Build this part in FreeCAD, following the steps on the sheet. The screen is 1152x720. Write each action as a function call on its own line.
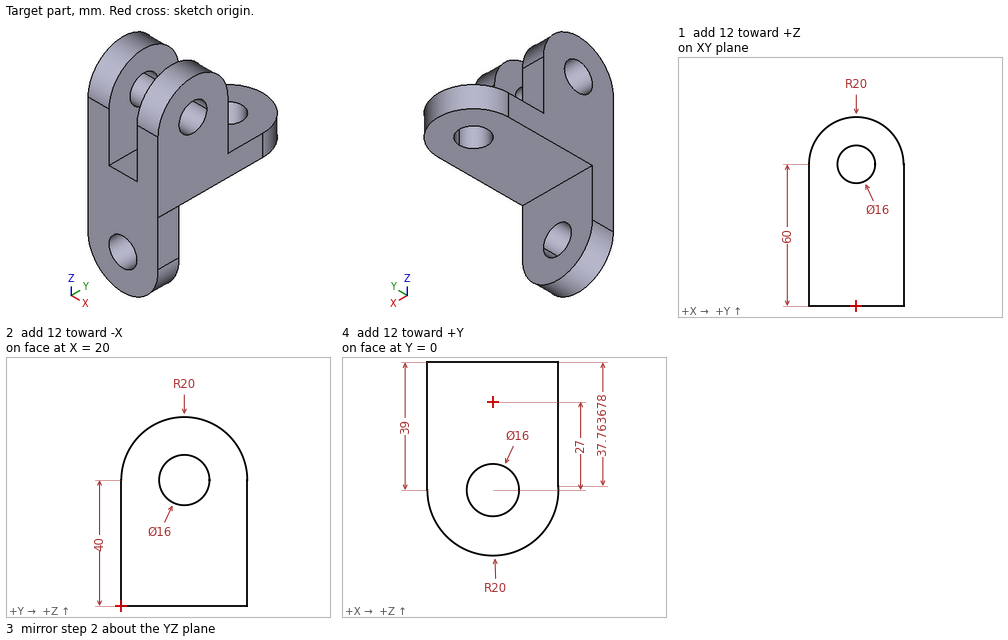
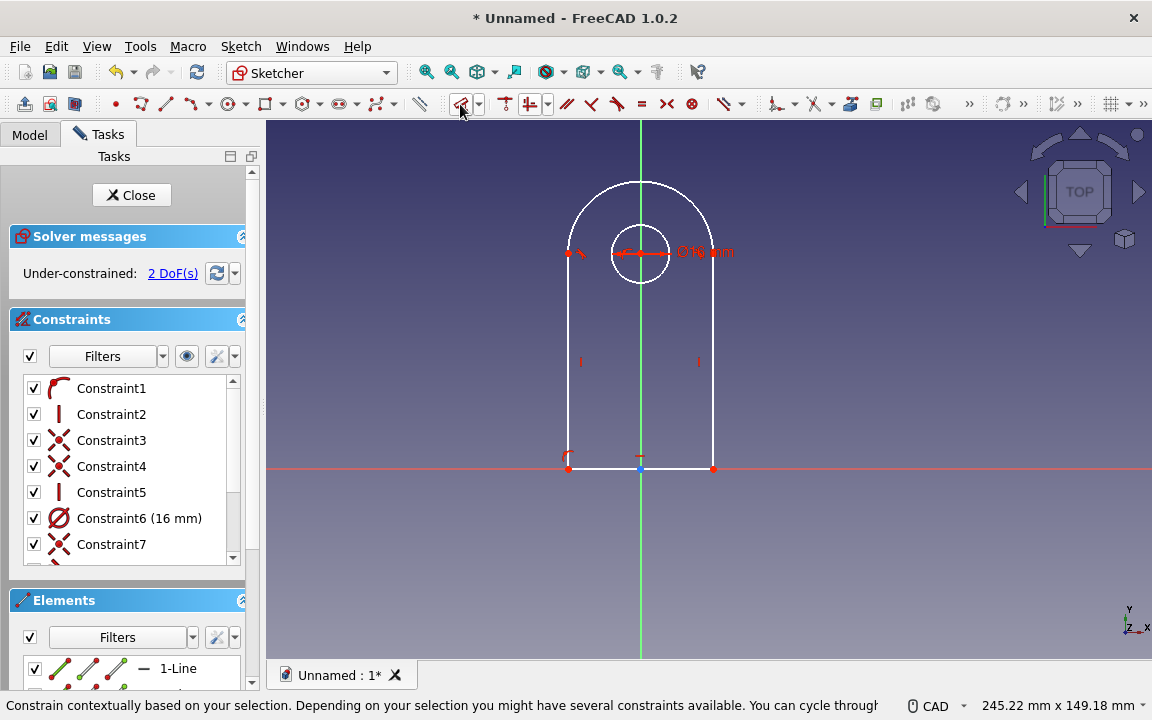
click(683, 195)
click(702, 169)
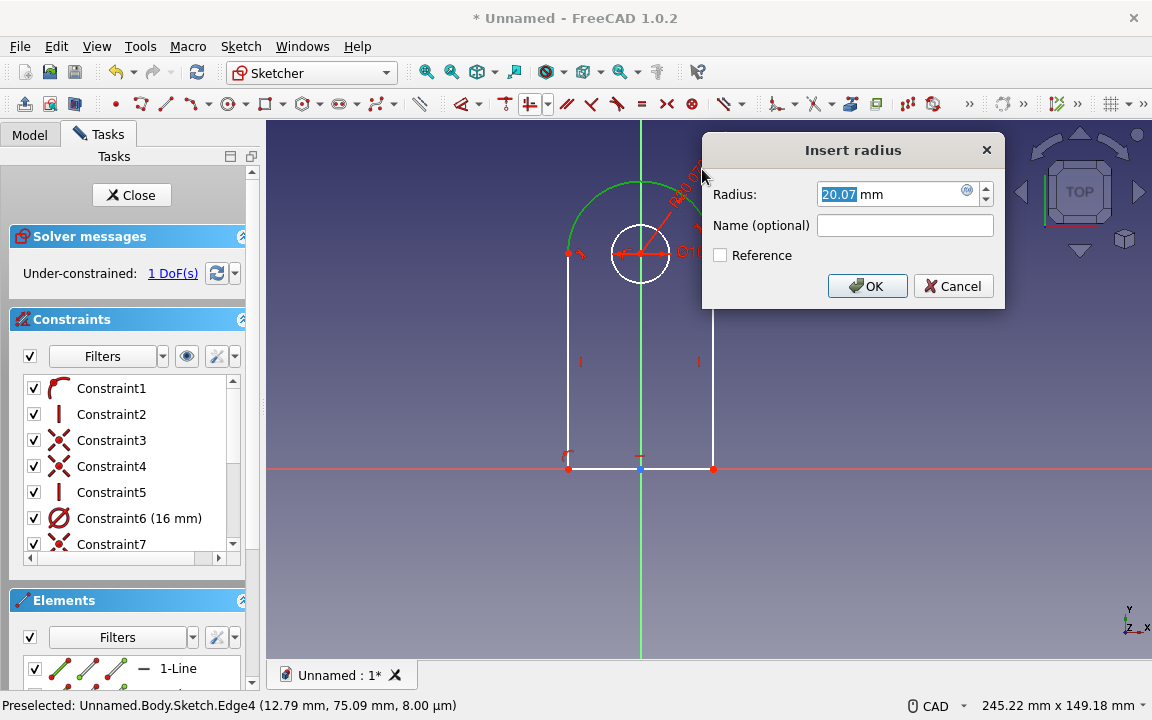
text(20)
key(Return)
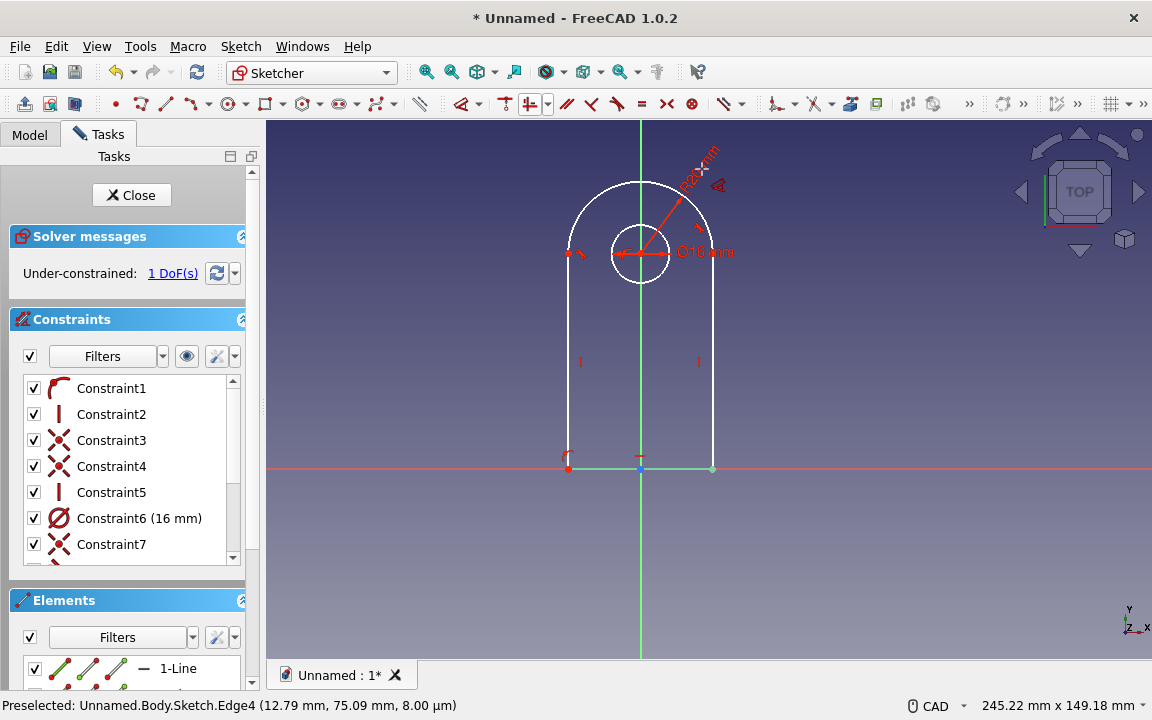
click(568, 319)
click(534, 362)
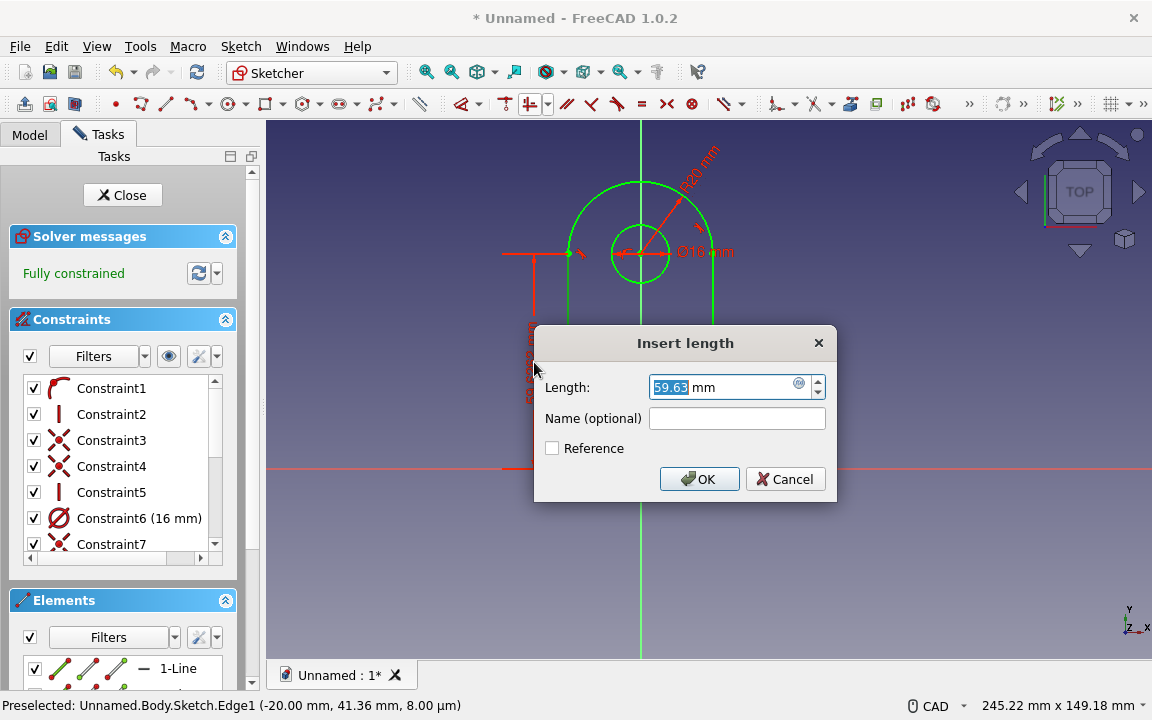
text(60)
key(Return)
key(Escape)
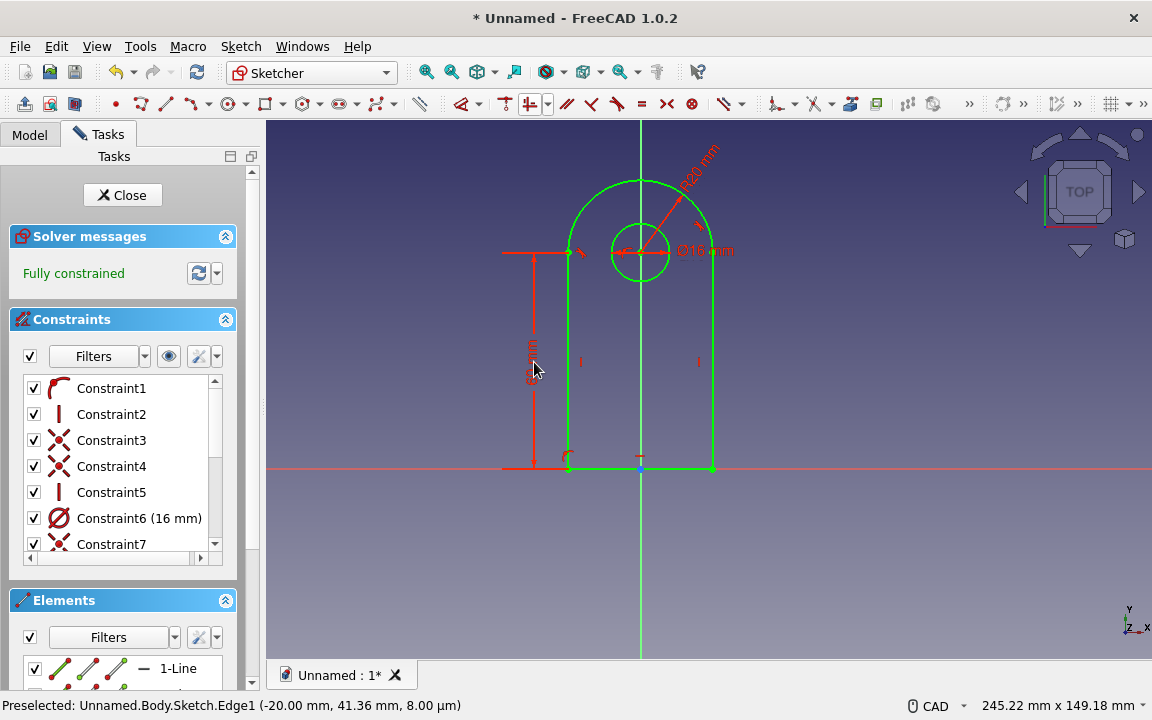
click(123, 195)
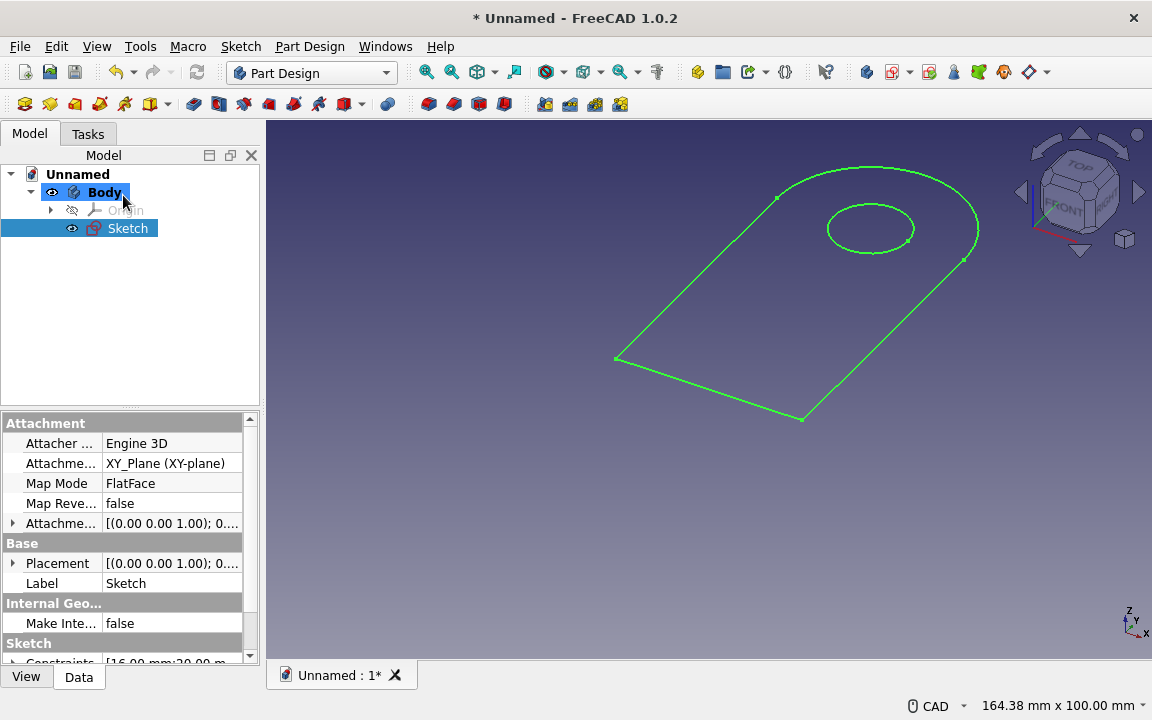
click(25, 104)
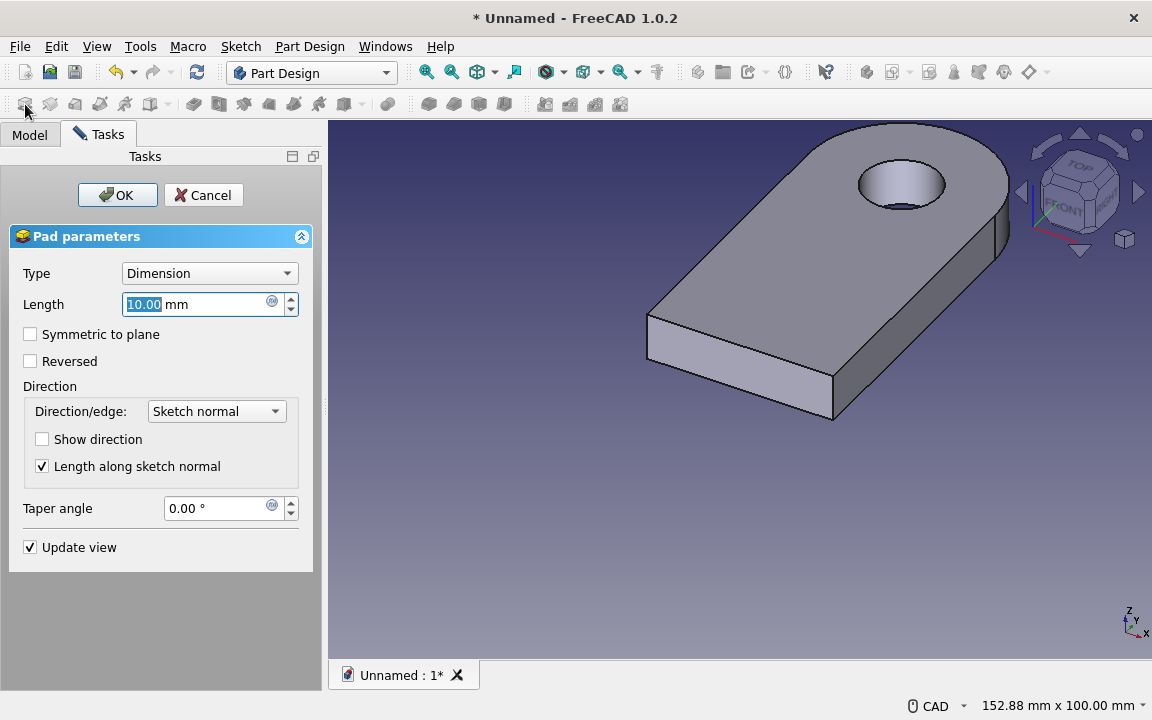
text(12)
key(Tab)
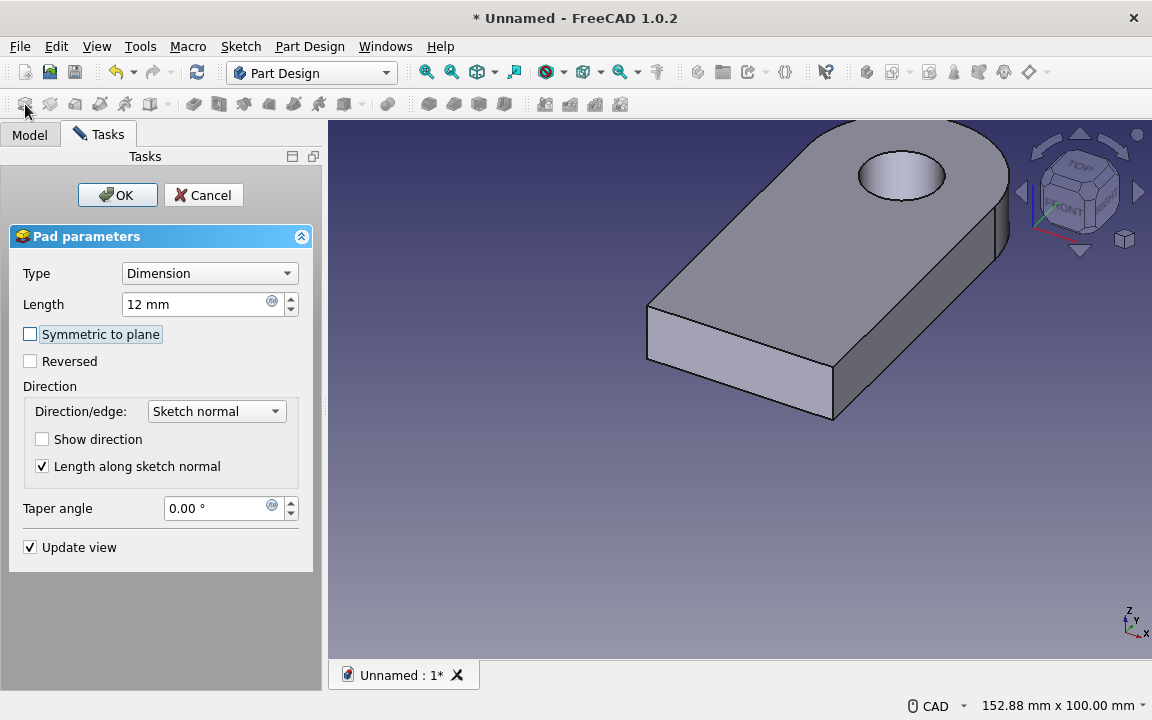
click(118, 195)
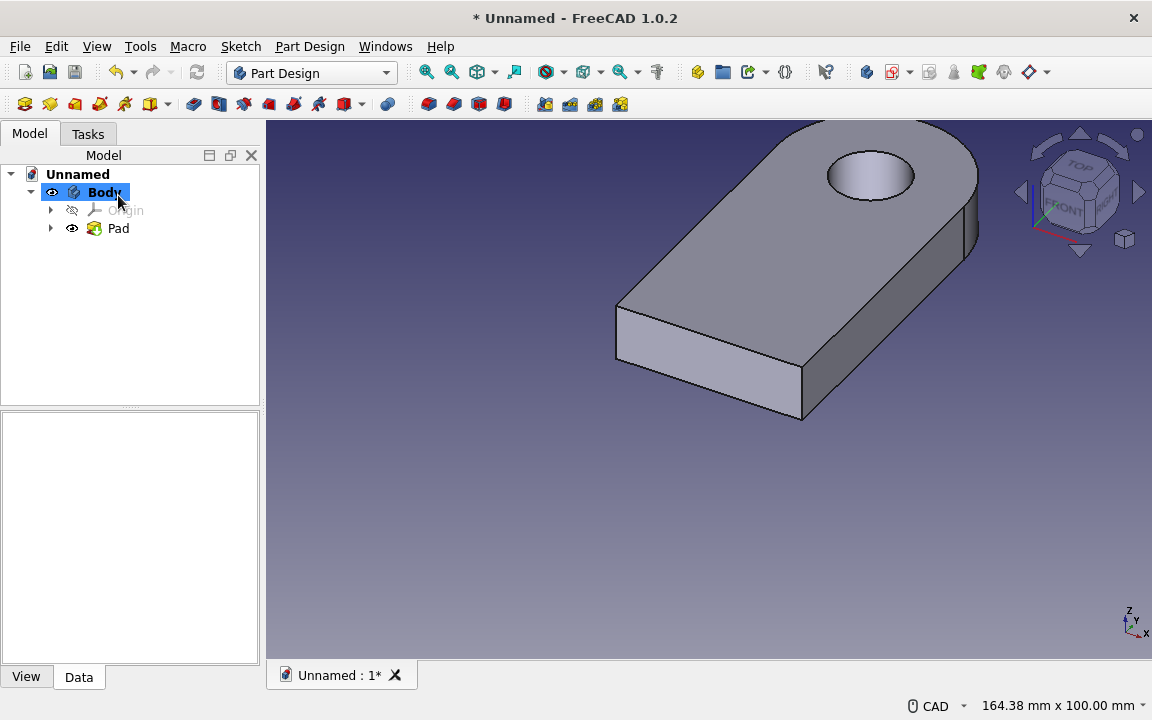
key(v)
key(f)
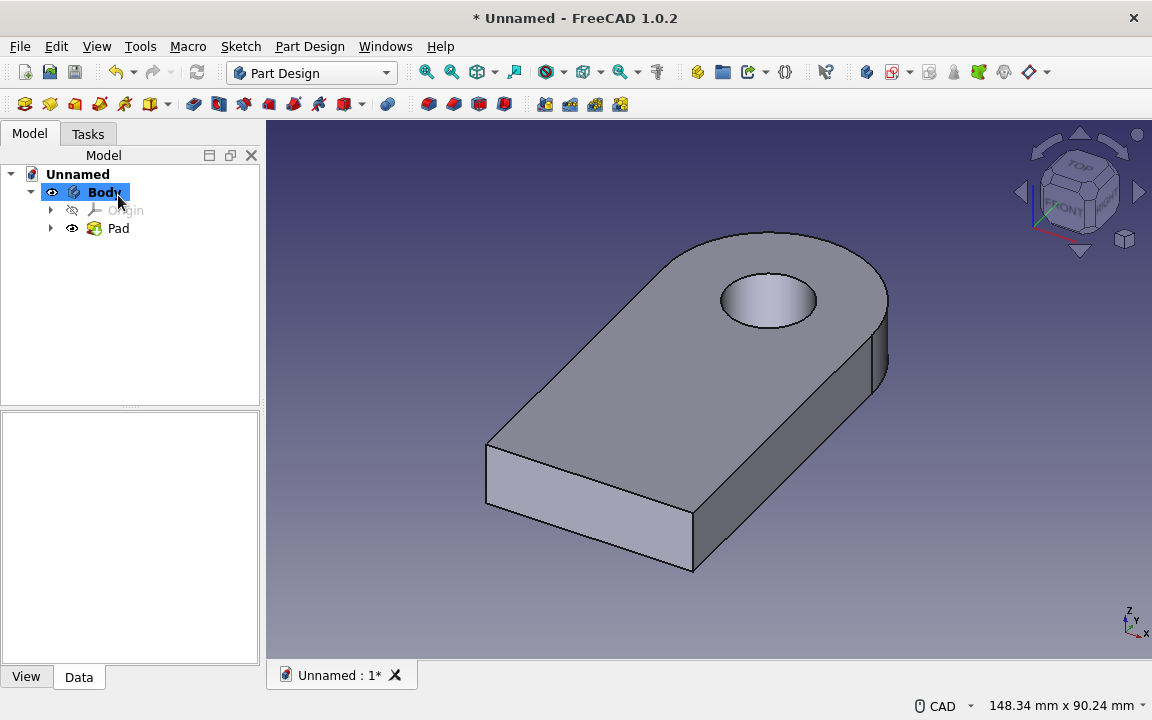
click(834, 402)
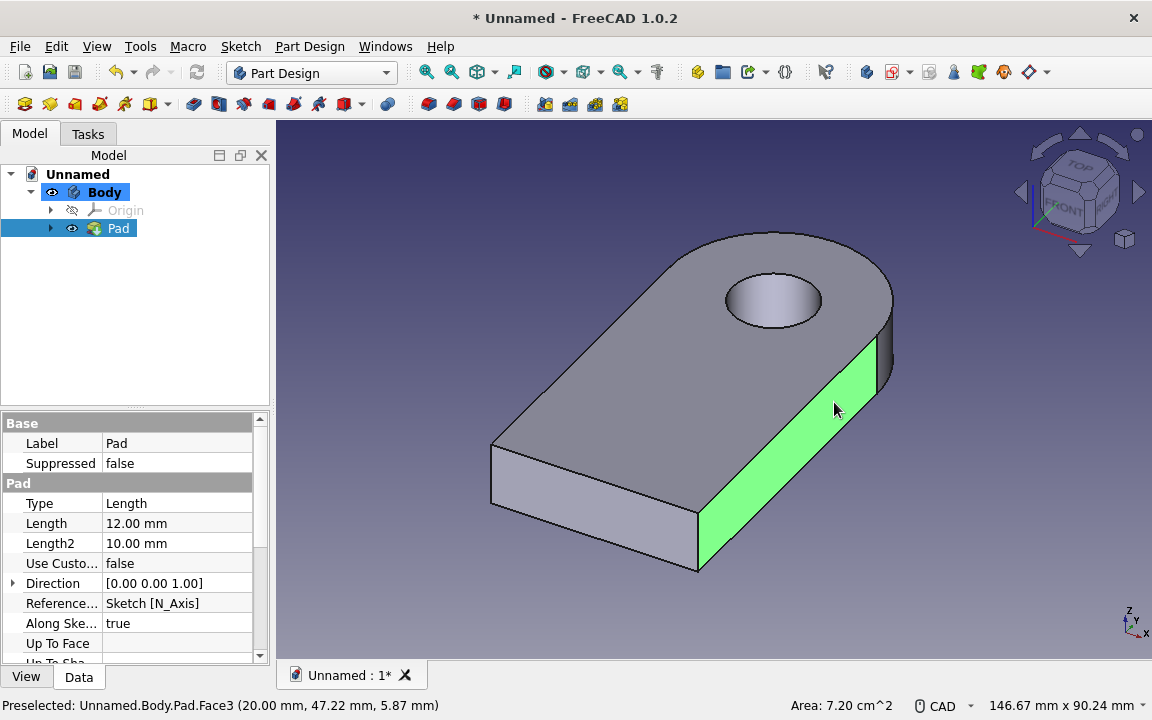
click(892, 72)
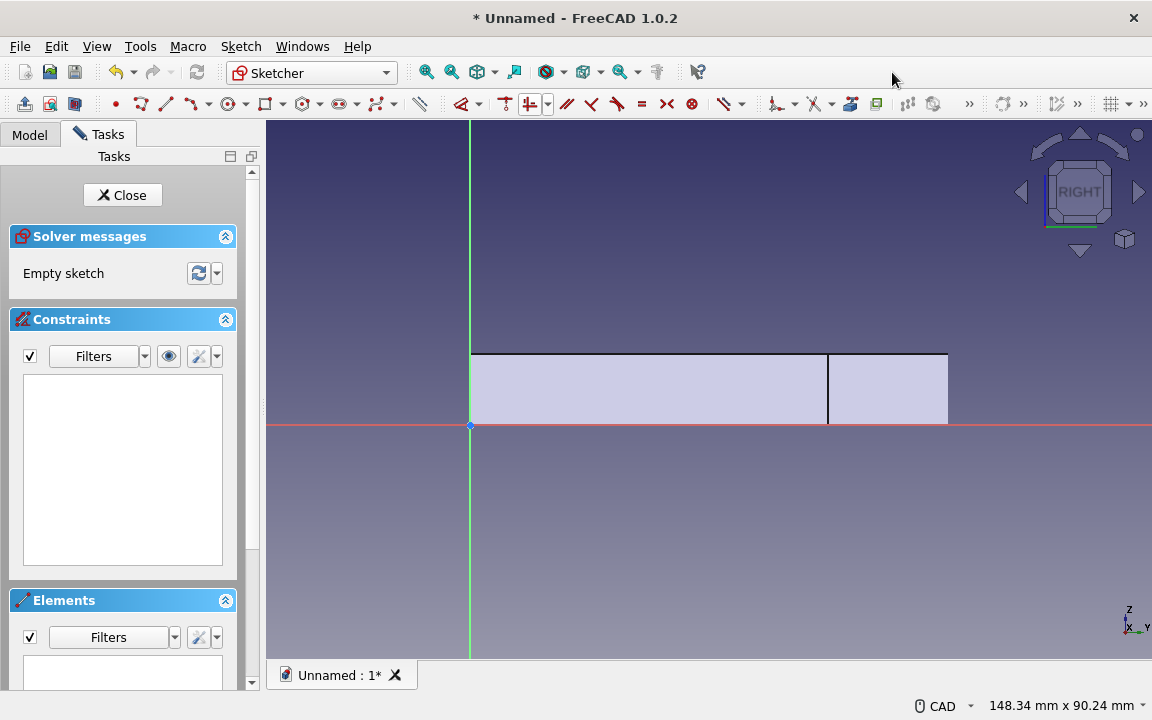
scroll(744, 631, down, 2)